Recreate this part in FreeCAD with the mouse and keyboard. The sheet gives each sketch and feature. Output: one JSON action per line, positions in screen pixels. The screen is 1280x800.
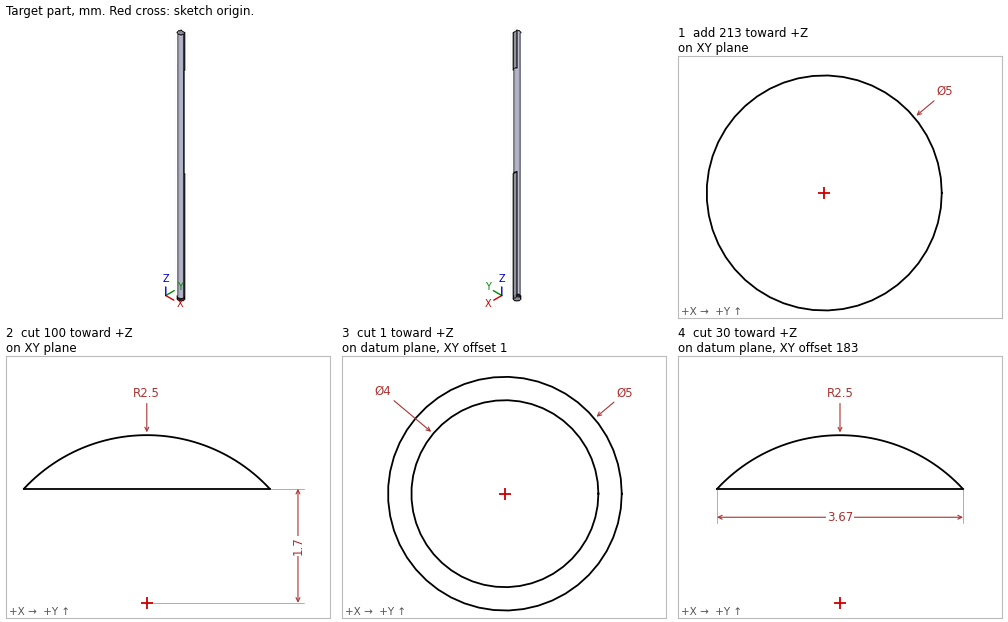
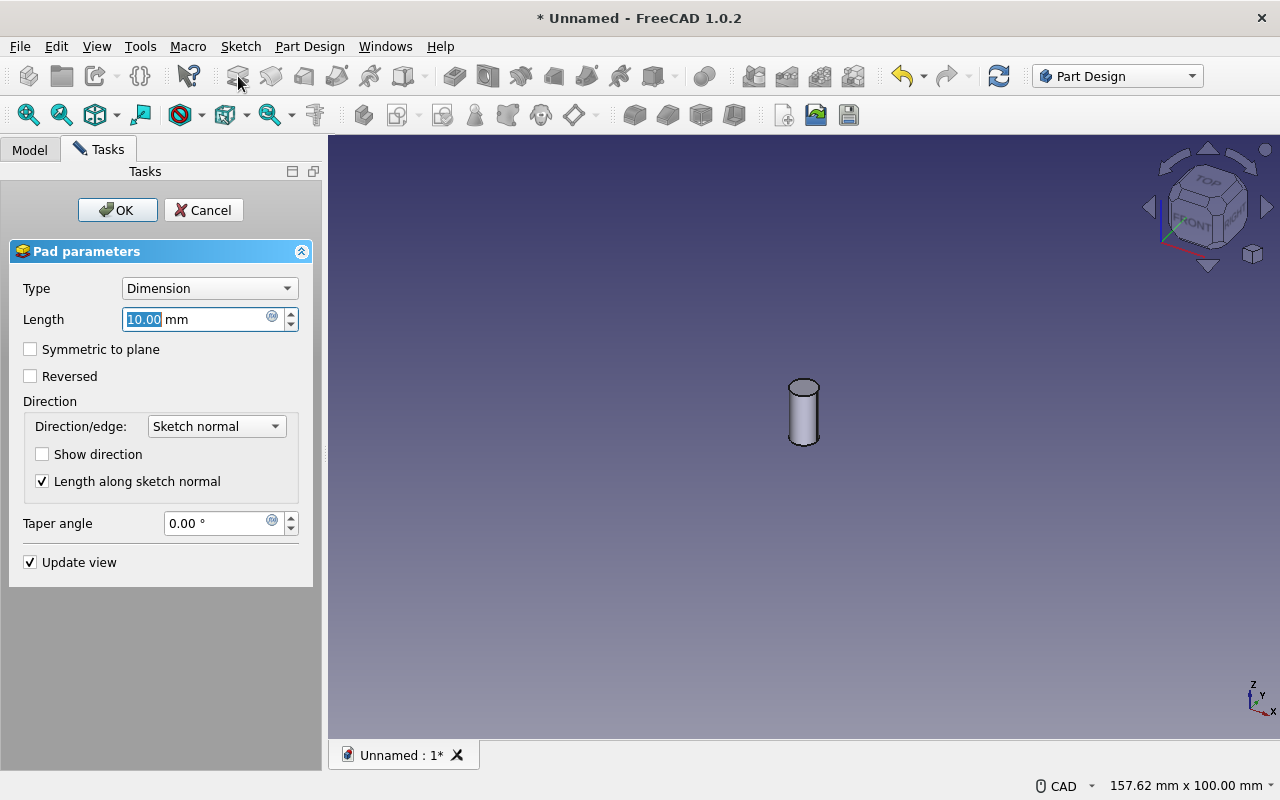
{"action": "type", "text": "213"}
{"action": "key", "text": "Tab"}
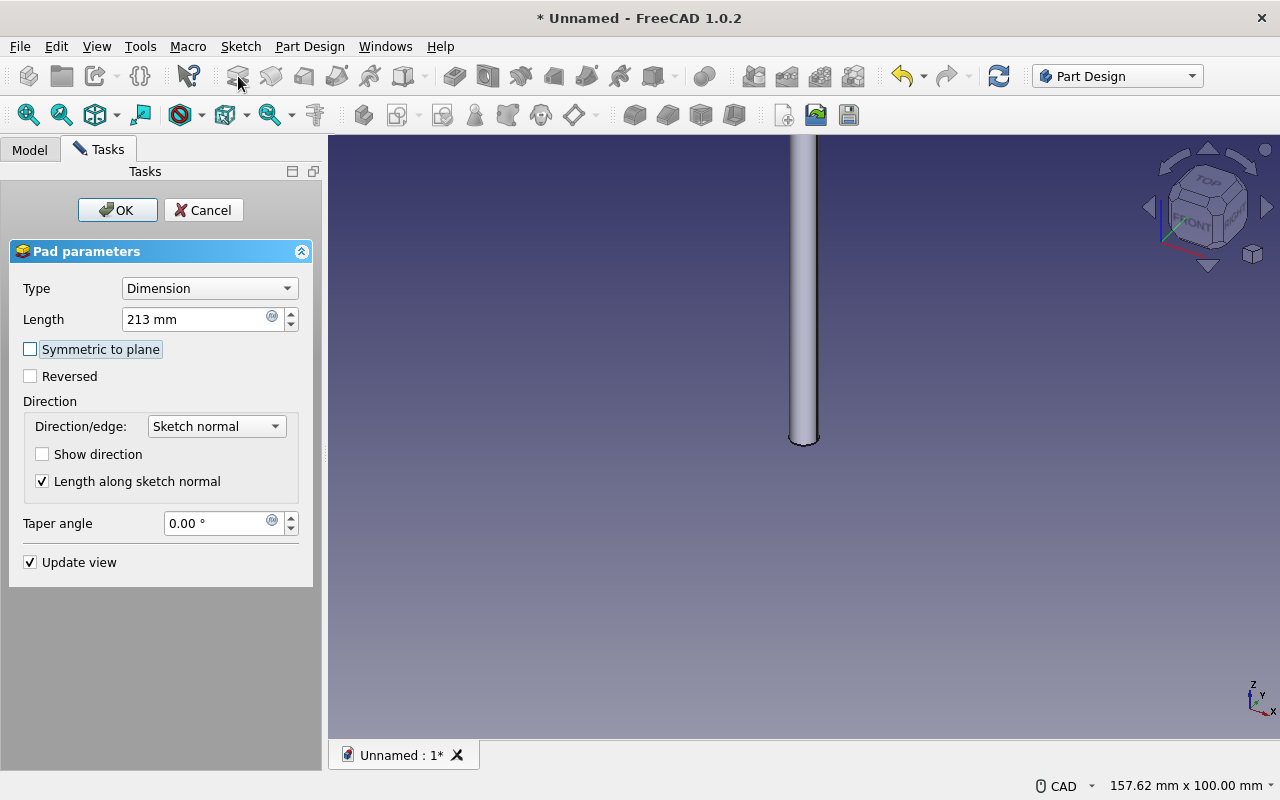
{"action": "left_click", "coordinate": [118, 210]}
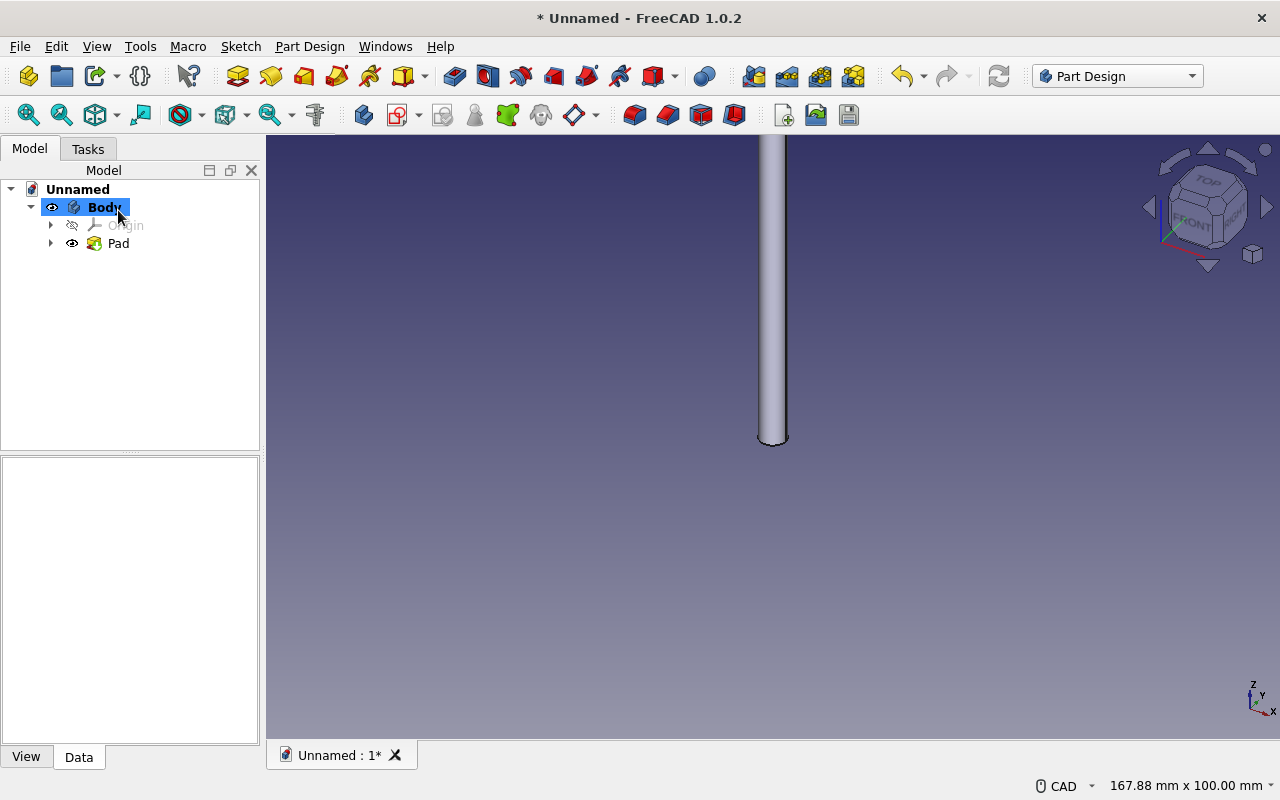
{"action": "key", "text": "v f"}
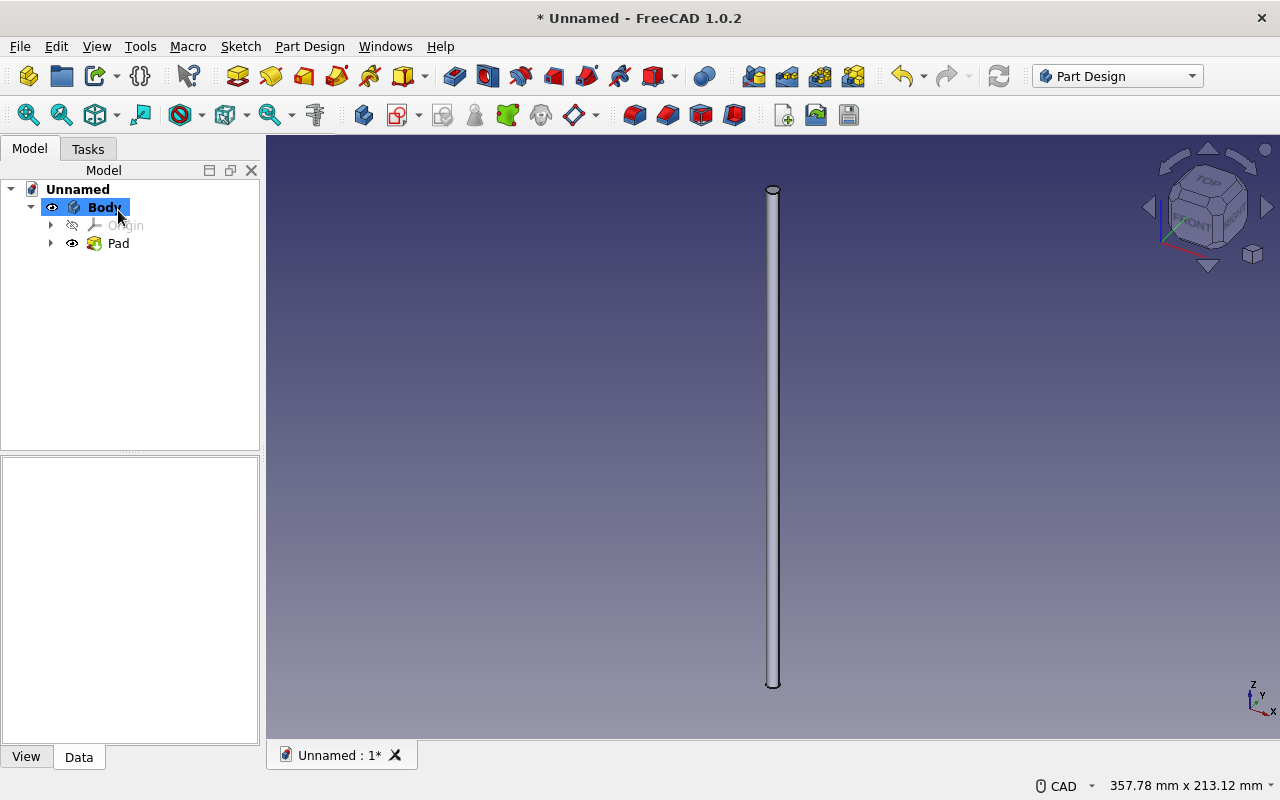
{"action": "left_click", "coordinate": [396, 116]}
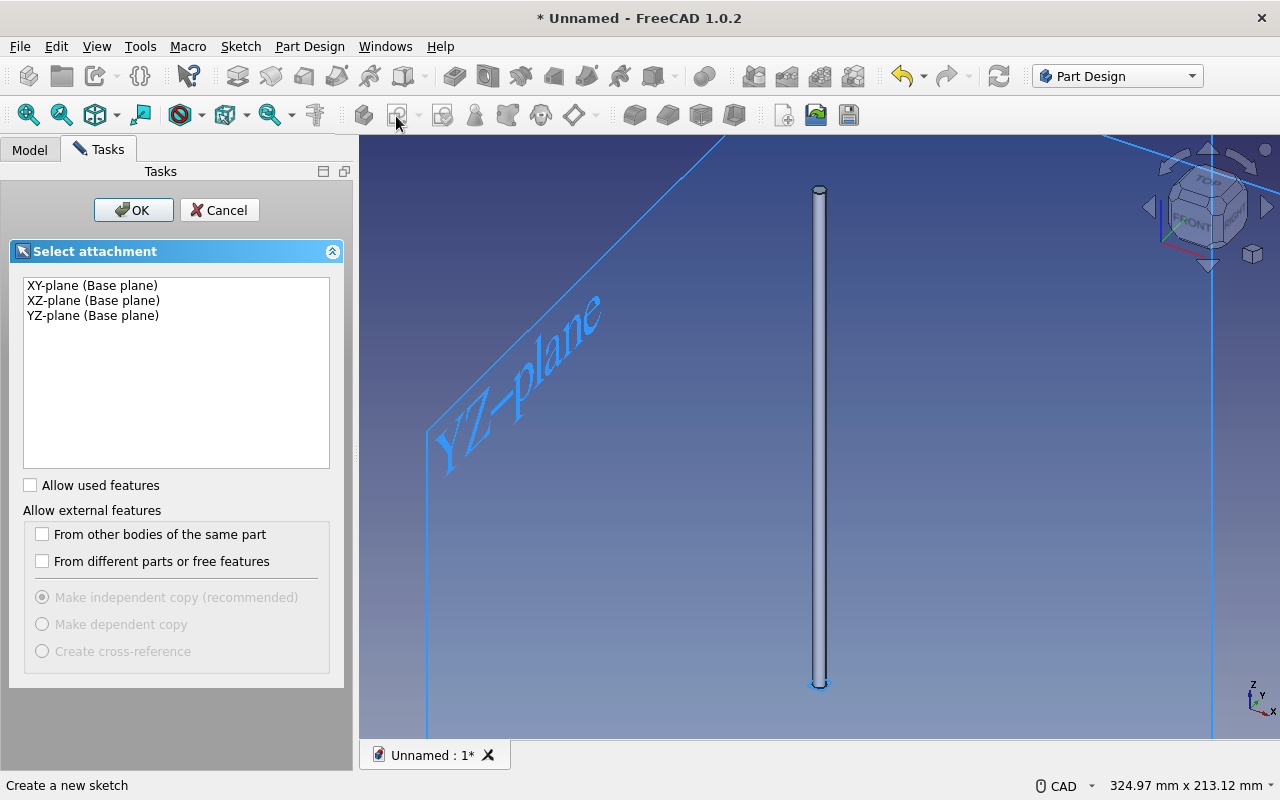
{"action": "left_click", "coordinate": [84, 286]}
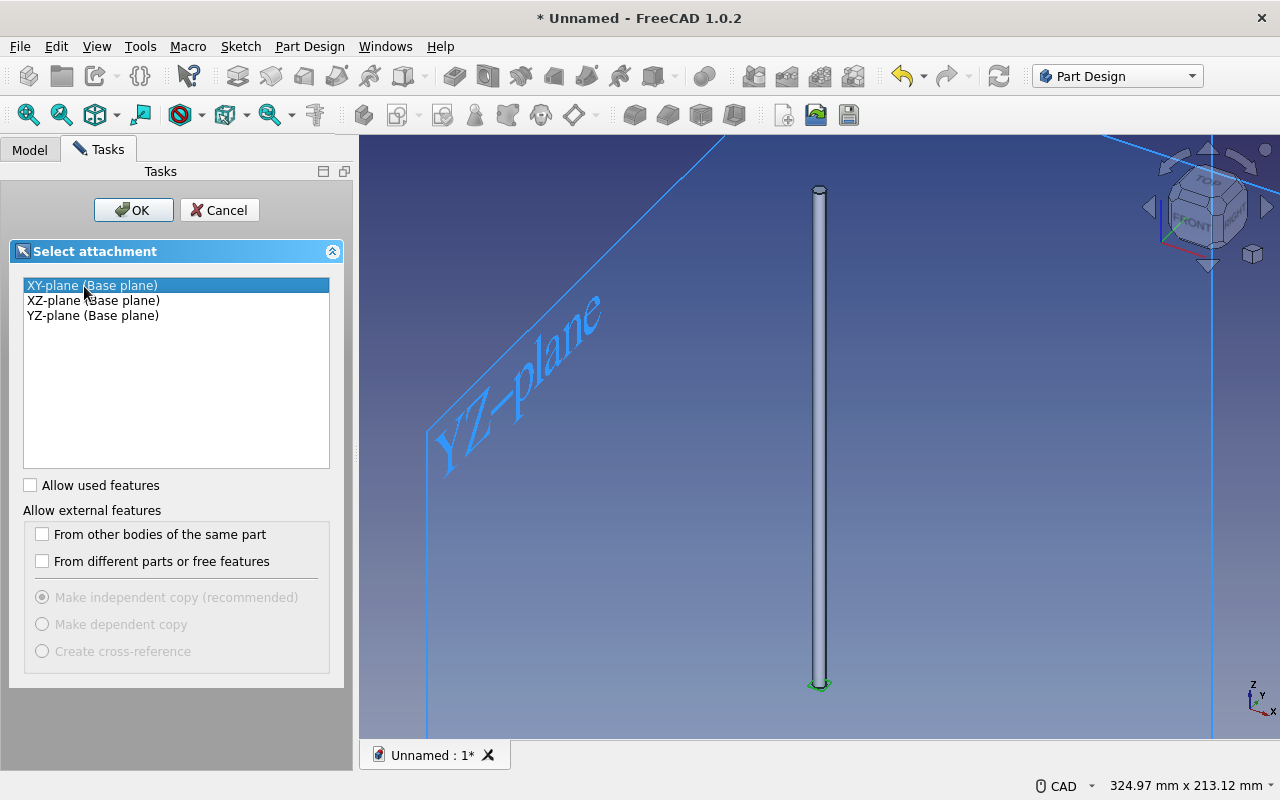
{"action": "left_click", "coordinate": [134, 210]}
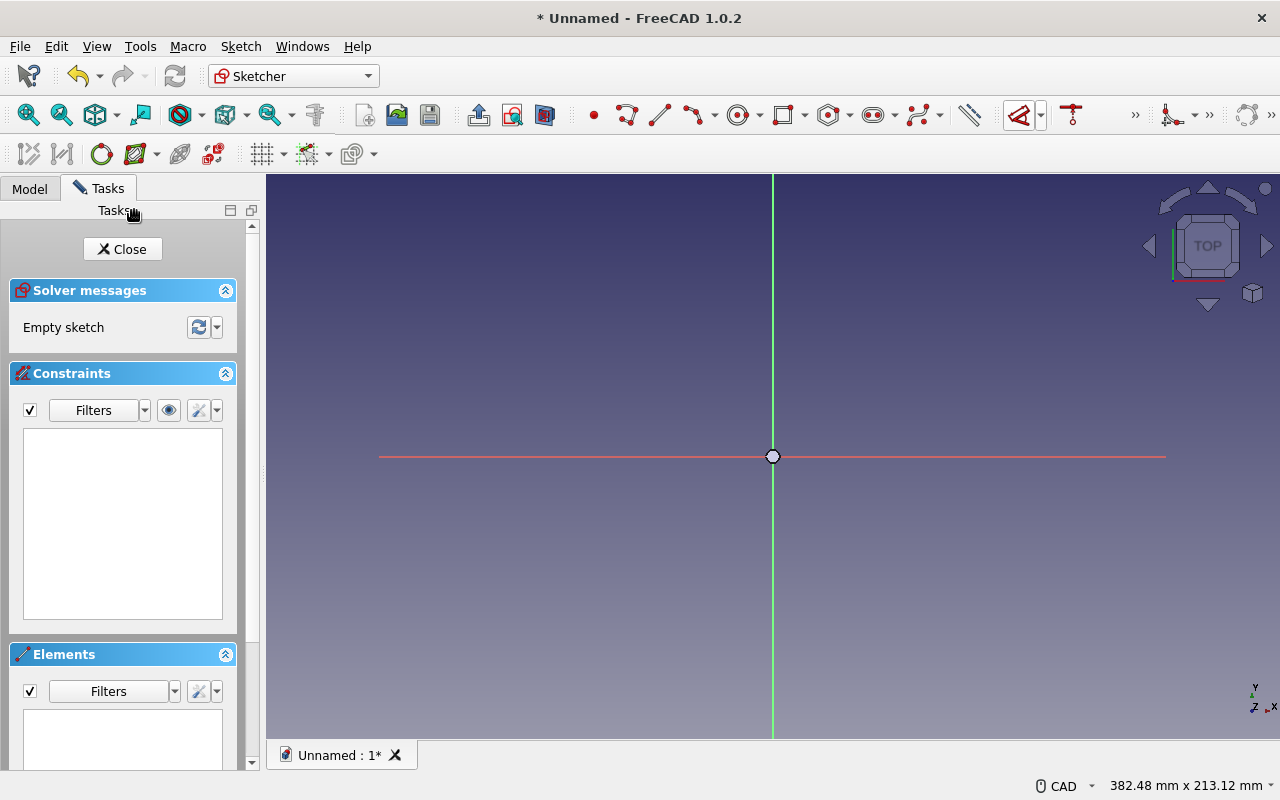
{"action": "key", "text": "q s"}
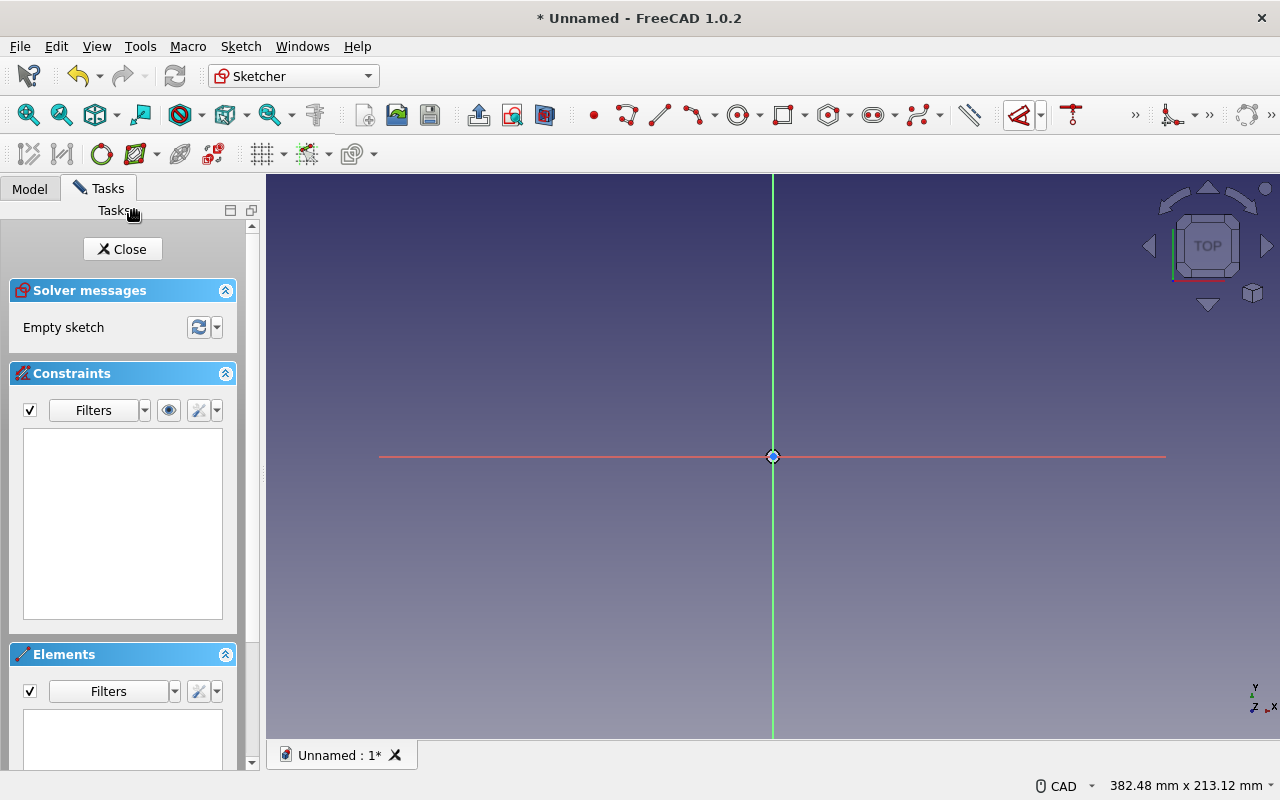
{"action": "scroll", "coordinate": [777, 453], "scroll_direction": "up", "scroll_amount": 15}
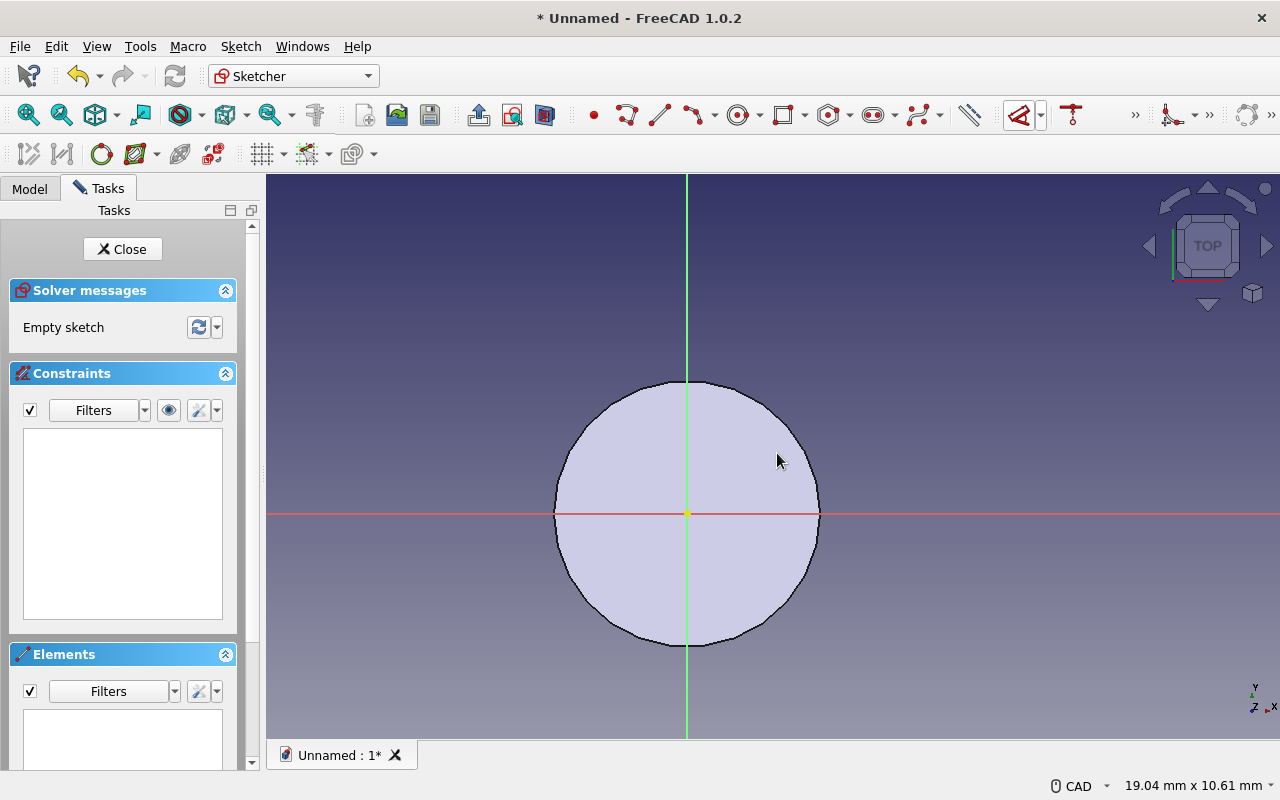
{"action": "scroll", "coordinate": [677, 442], "scroll_direction": "up", "scroll_amount": 5}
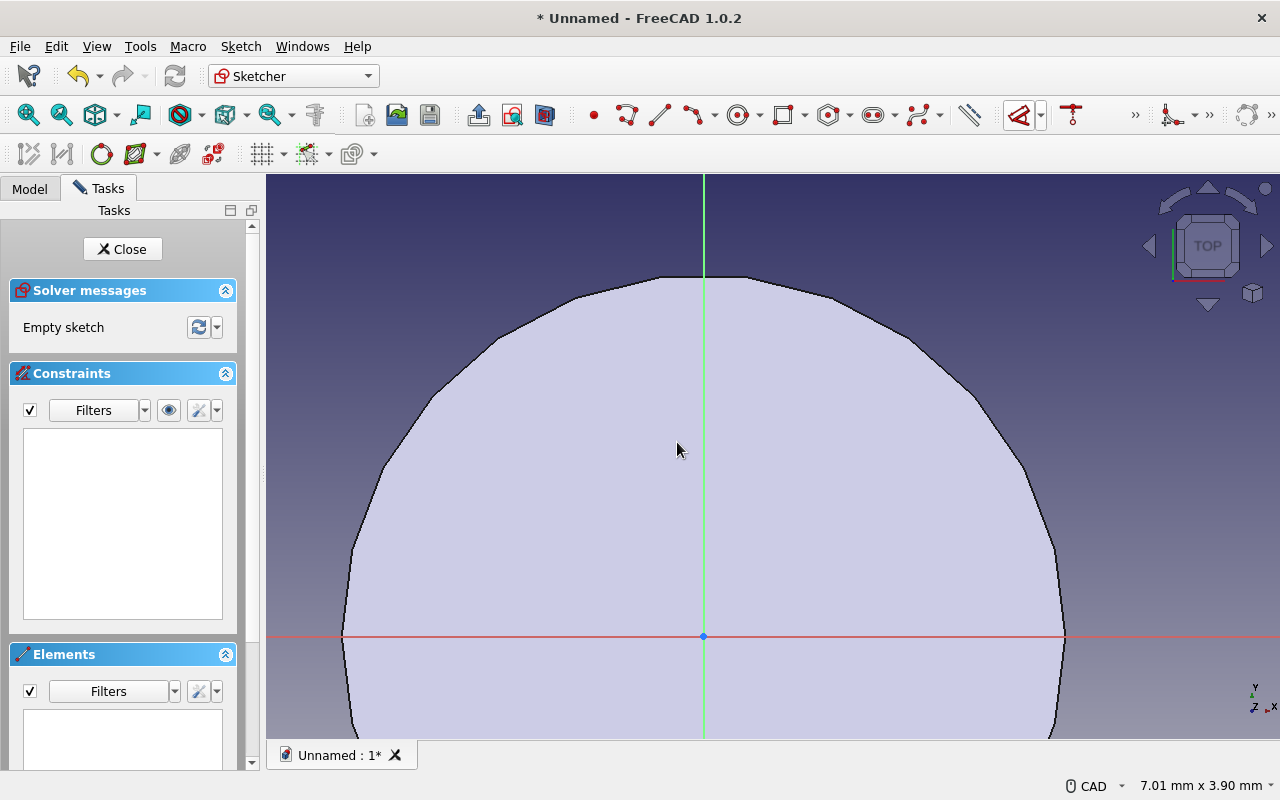
{"action": "key", "text": "g l"}